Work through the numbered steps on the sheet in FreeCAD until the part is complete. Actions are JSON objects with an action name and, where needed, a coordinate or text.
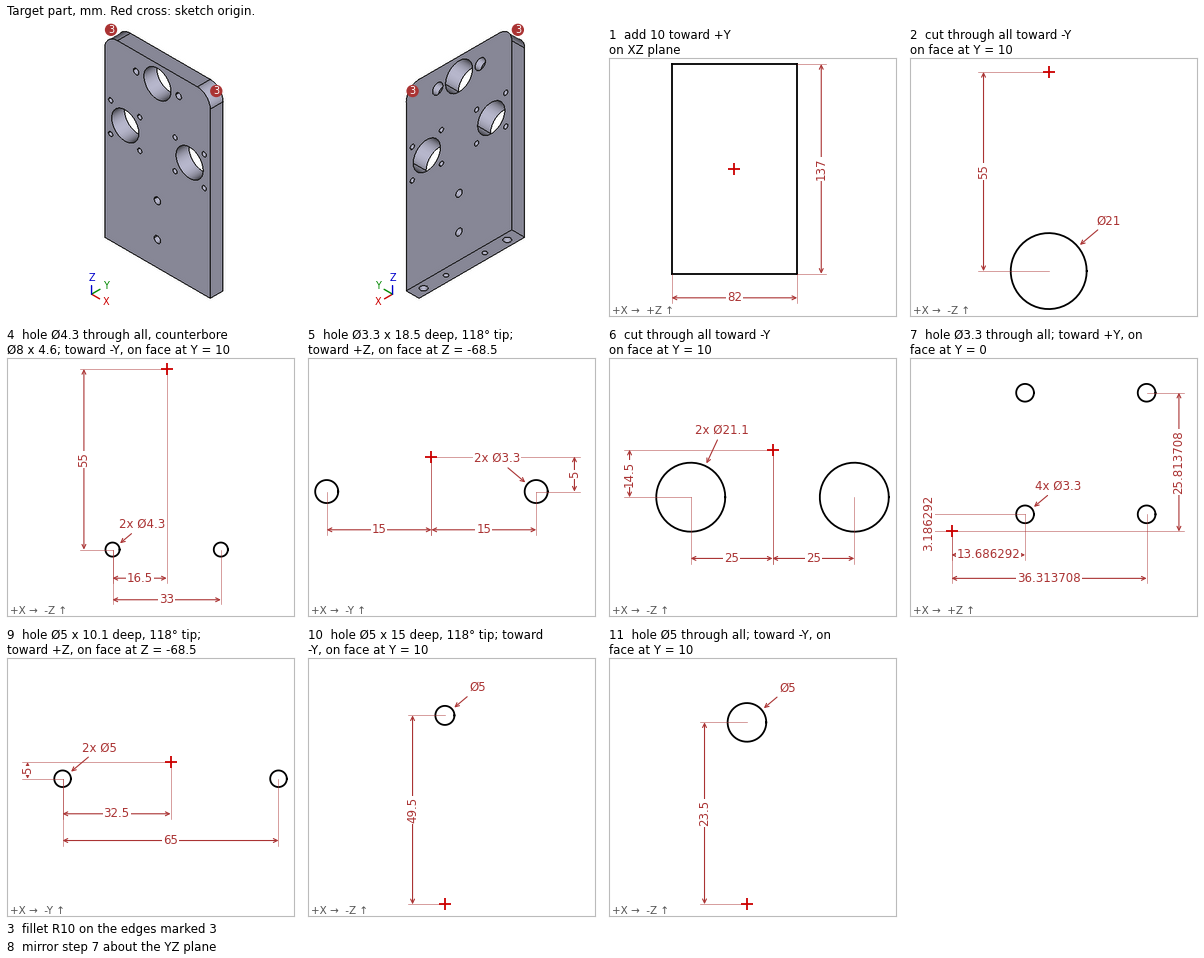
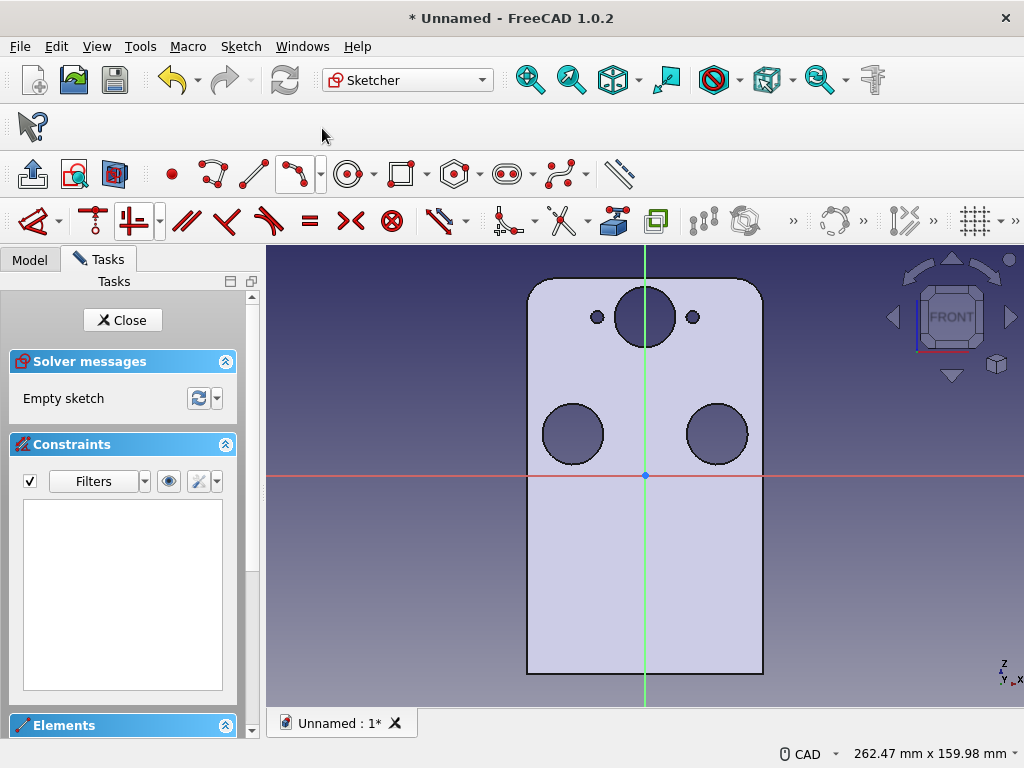
{"action": "scroll", "coordinate": [753, 419], "scroll_direction": "up", "scroll_amount": 6}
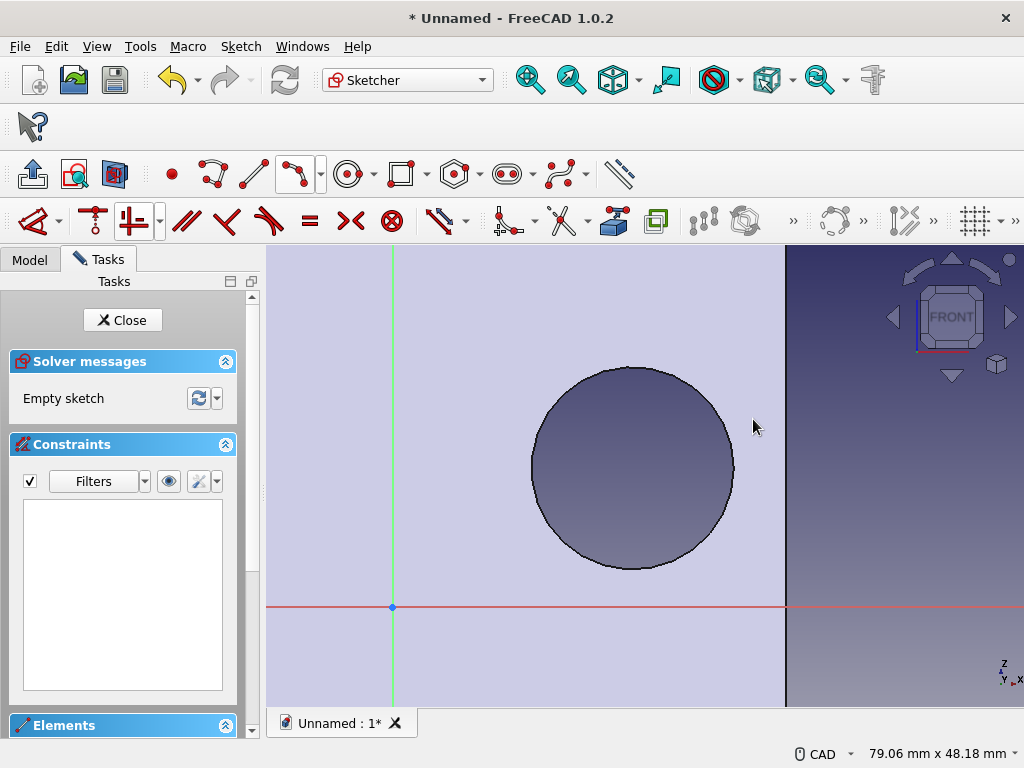
{"action": "key", "text": "g c"}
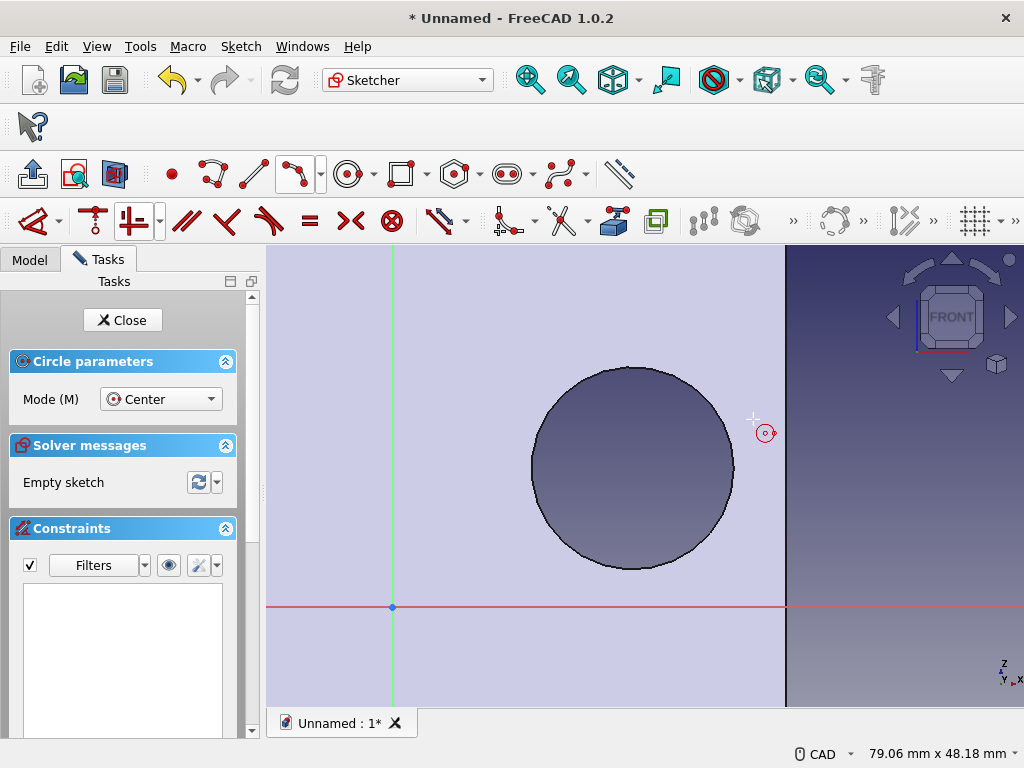
{"action": "scroll", "coordinate": [524, 577], "scroll_direction": "up", "scroll_amount": 2}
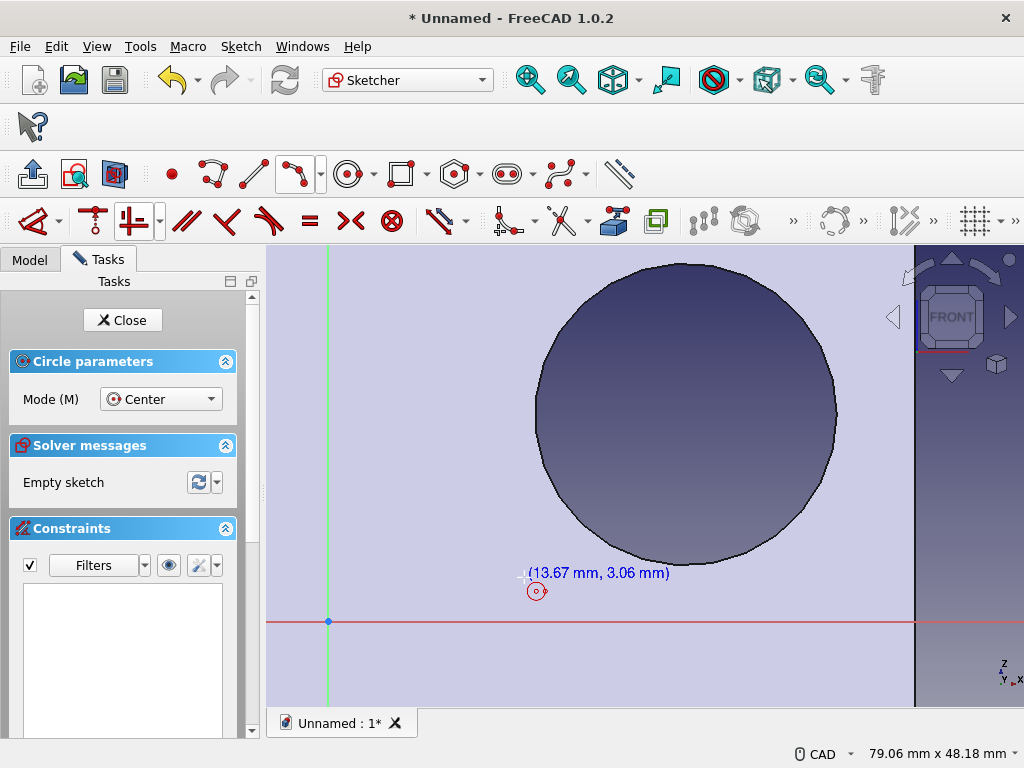
{"action": "left_click", "coordinate": [524, 576]}
{"action": "mouse_move", "coordinate": [541, 560]}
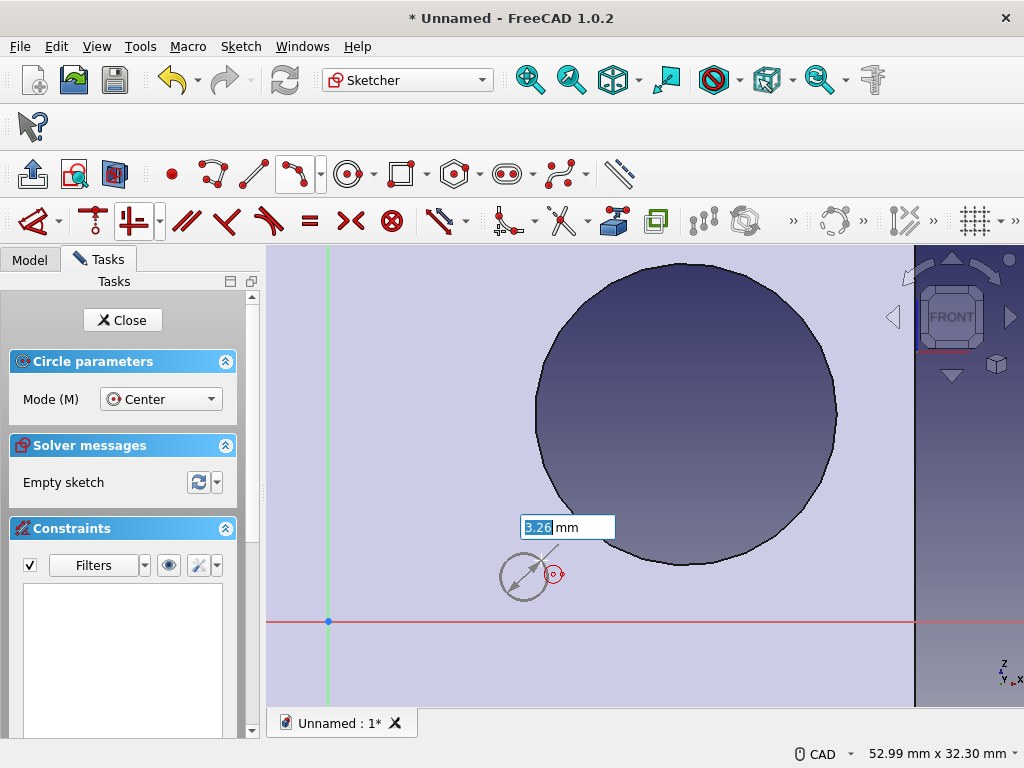
{"action": "type", "text": "3.3"}
{"action": "key", "text": "Return"}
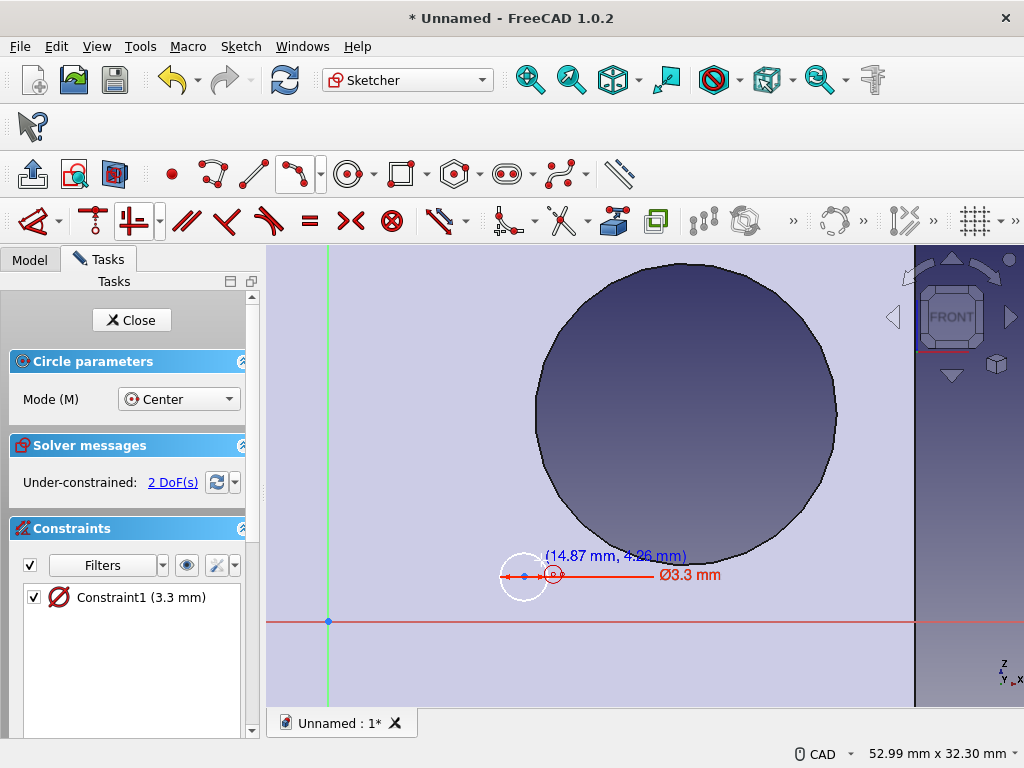
{"action": "left_click", "coordinate": [848, 576]}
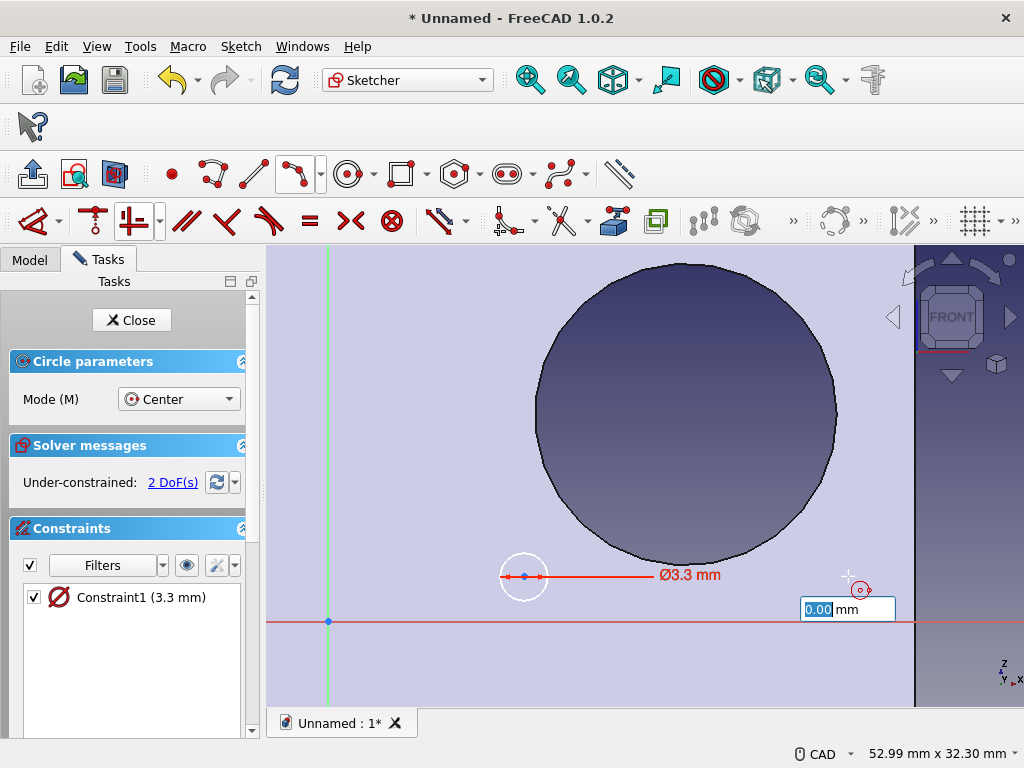
{"action": "scroll", "coordinate": [529, 579], "scroll_direction": "down", "scroll_amount": 2}
{"action": "mouse_move", "coordinate": [754, 566]}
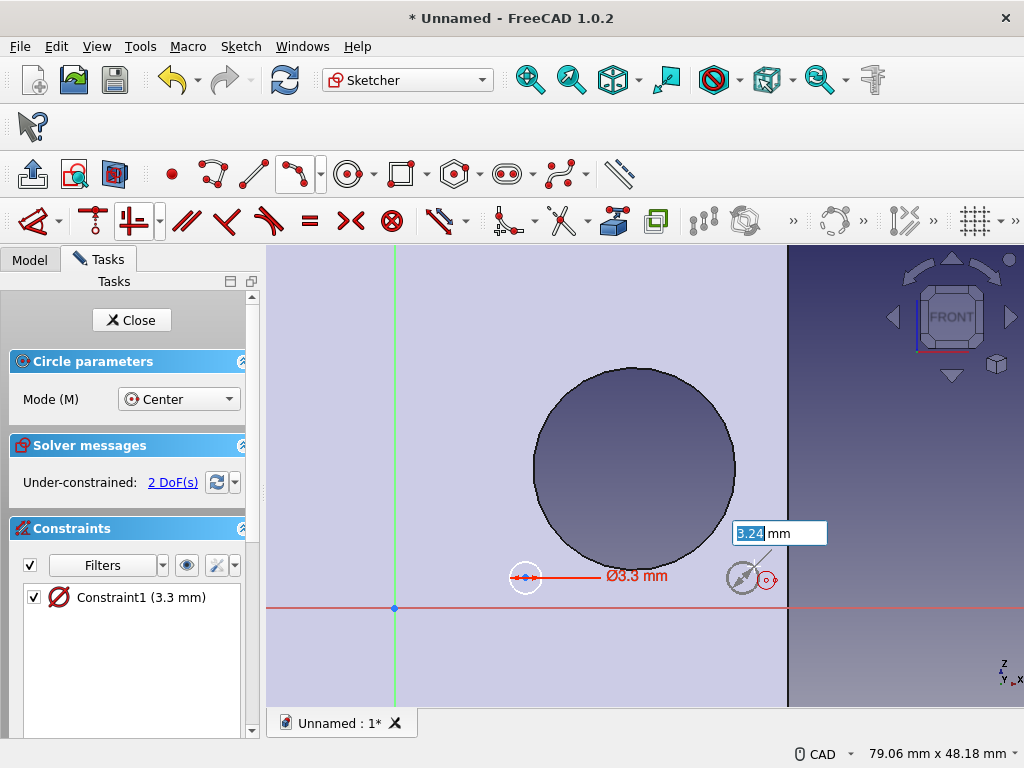
{"action": "type", "text": "3.3"}
{"action": "key", "text": "Return"}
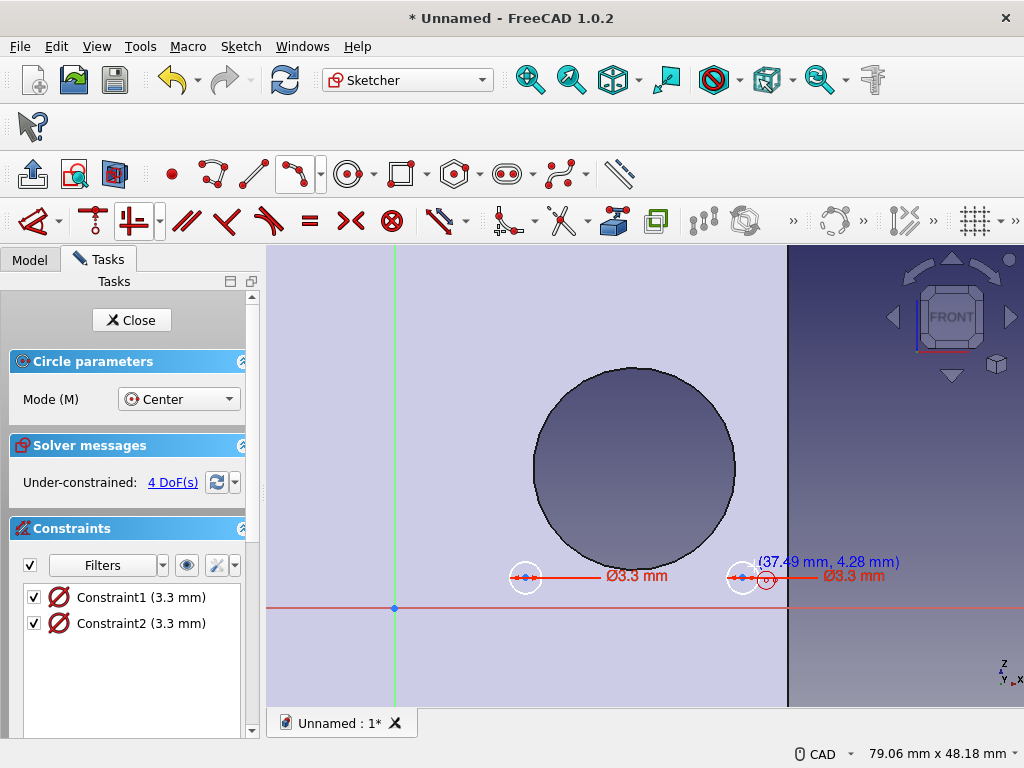
{"action": "scroll", "coordinate": [743, 361], "scroll_direction": "up", "scroll_amount": 2}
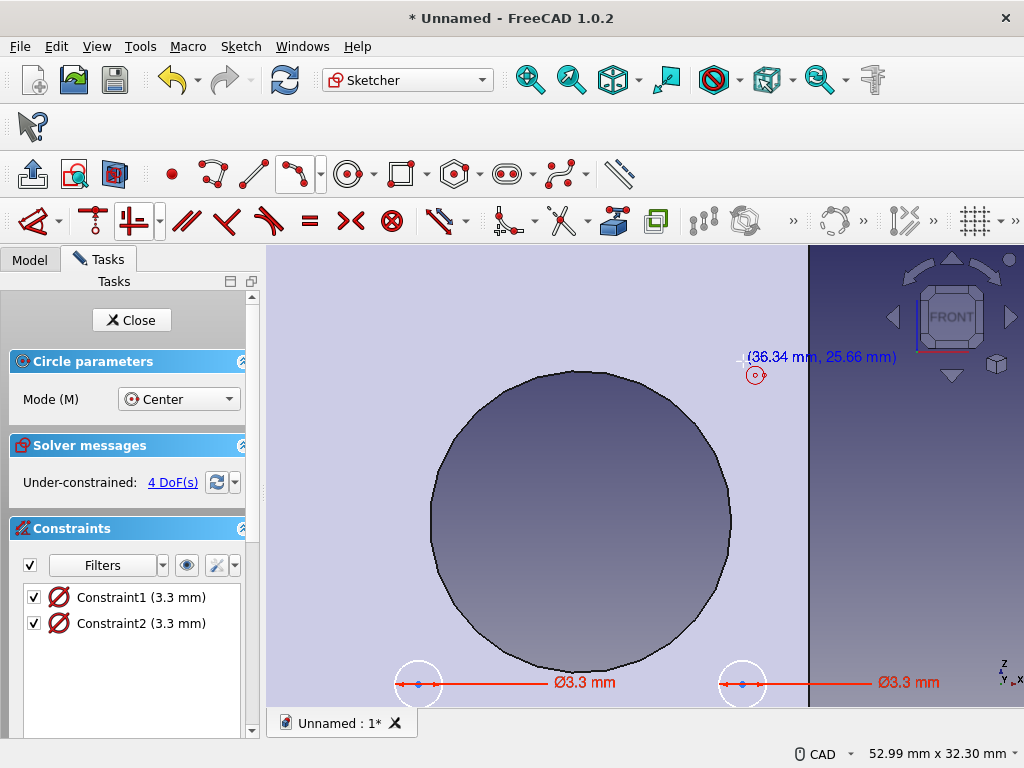
{"action": "left_click", "coordinate": [742, 360]}
{"action": "mouse_move", "coordinate": [759, 343]}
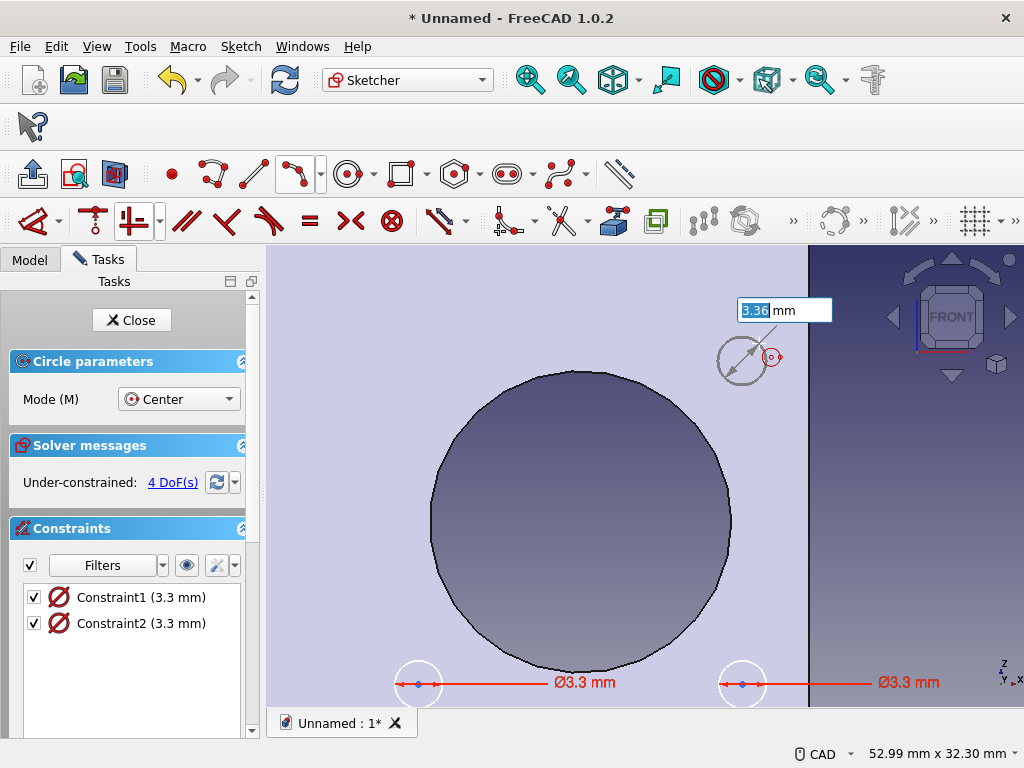
{"action": "type", "text": "3.3"}
{"action": "key", "text": "Return"}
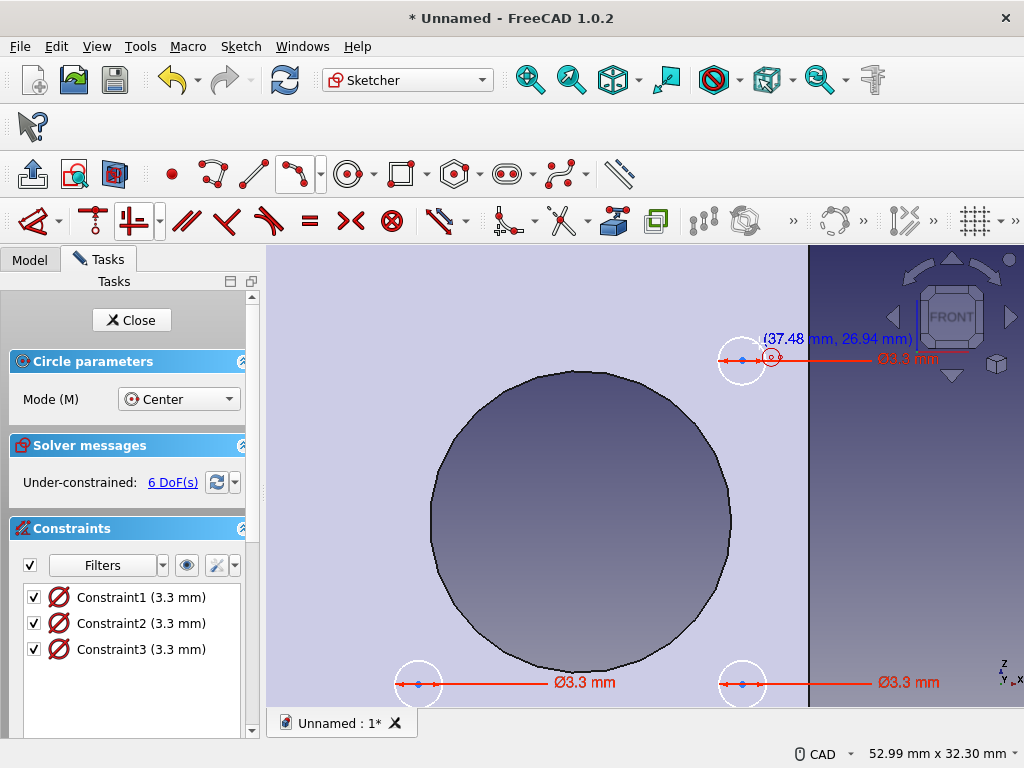
{"action": "left_click", "coordinate": [419, 360]}
{"action": "mouse_move", "coordinate": [435, 343]}